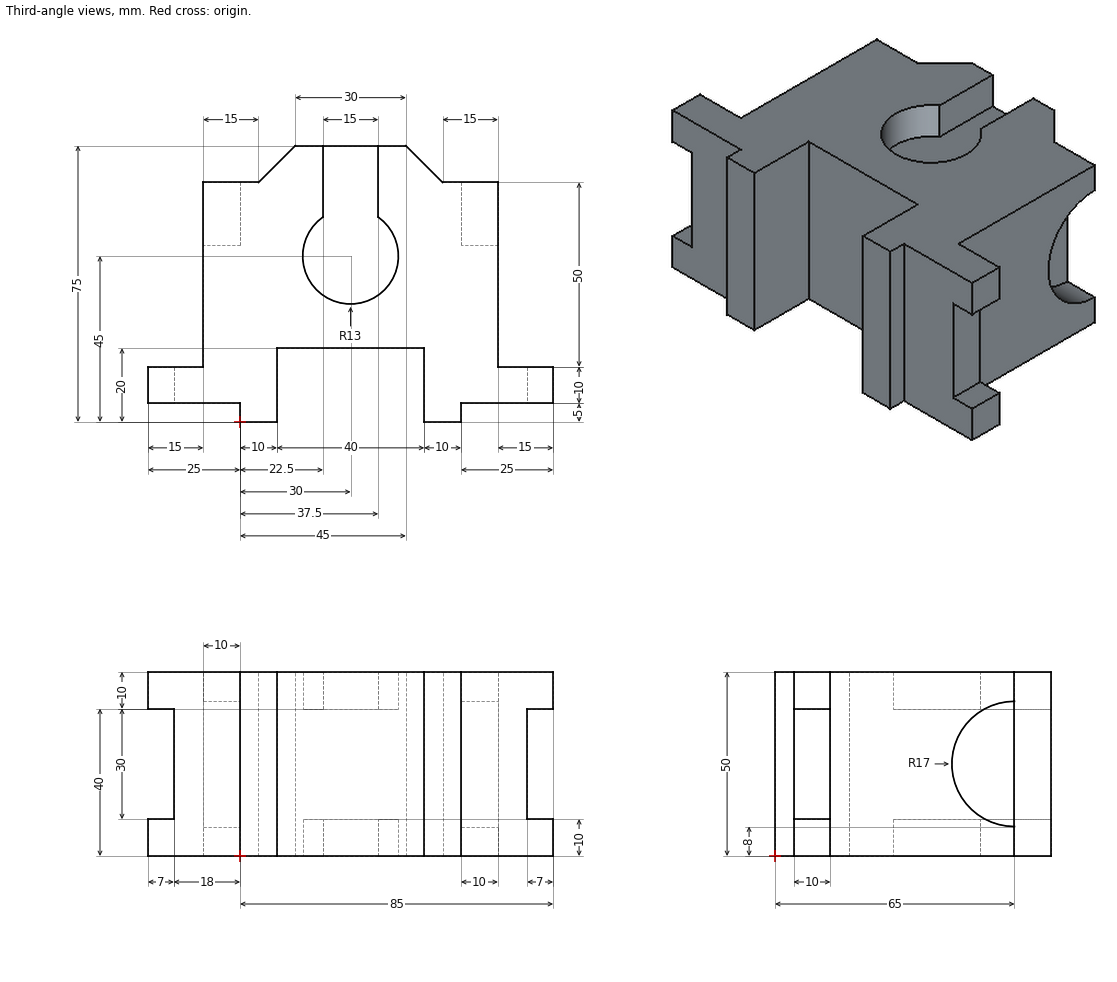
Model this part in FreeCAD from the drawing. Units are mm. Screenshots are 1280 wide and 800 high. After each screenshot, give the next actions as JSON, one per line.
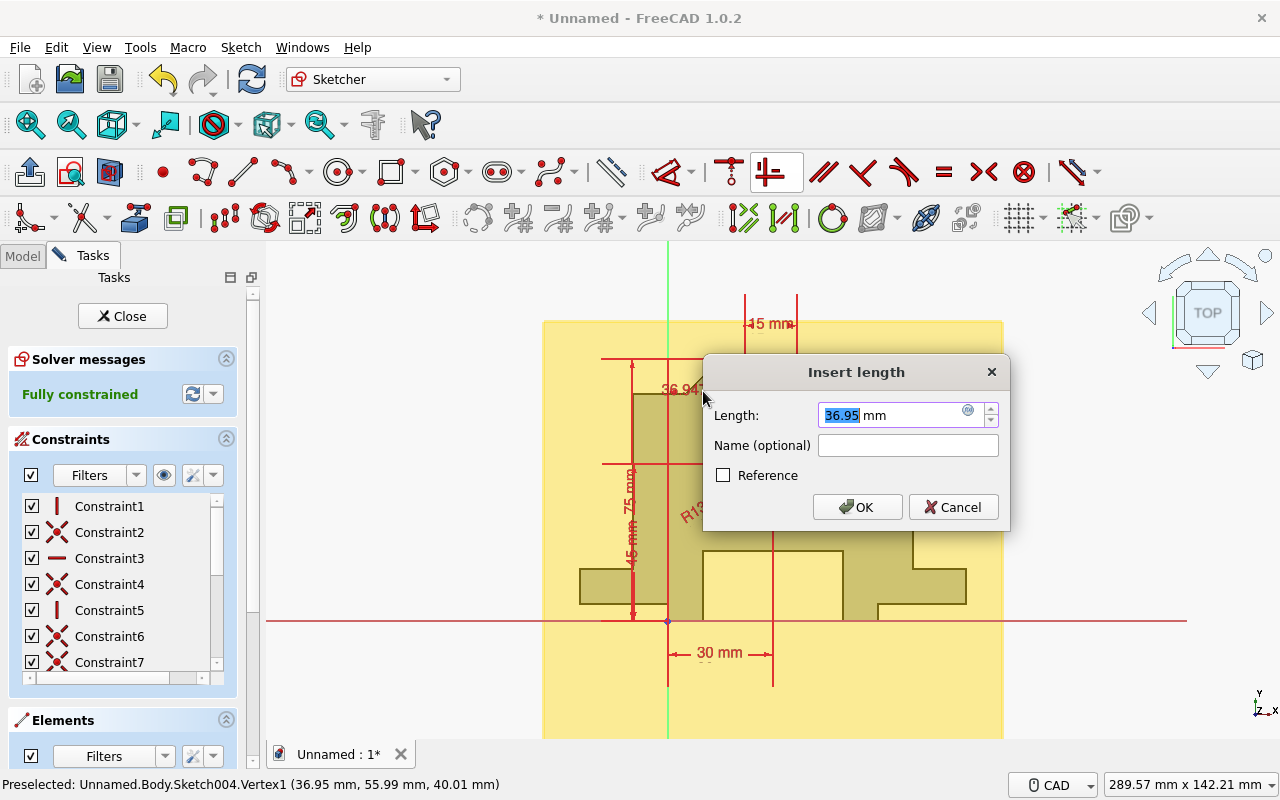
{"action": "type", "text": "37.5"}
{"action": "key", "text": "Return"}
{"action": "key", "text": "Escape"}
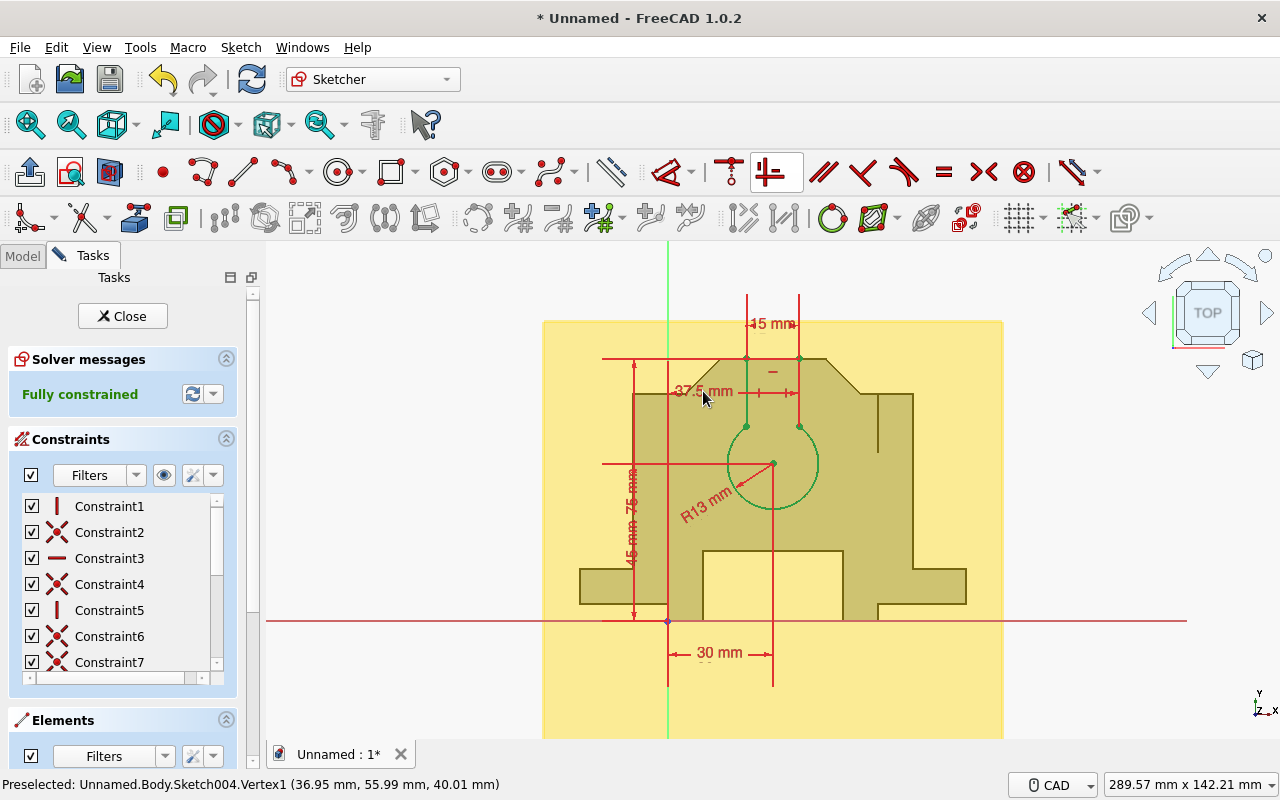
{"action": "left_click", "coordinate": [123, 316]}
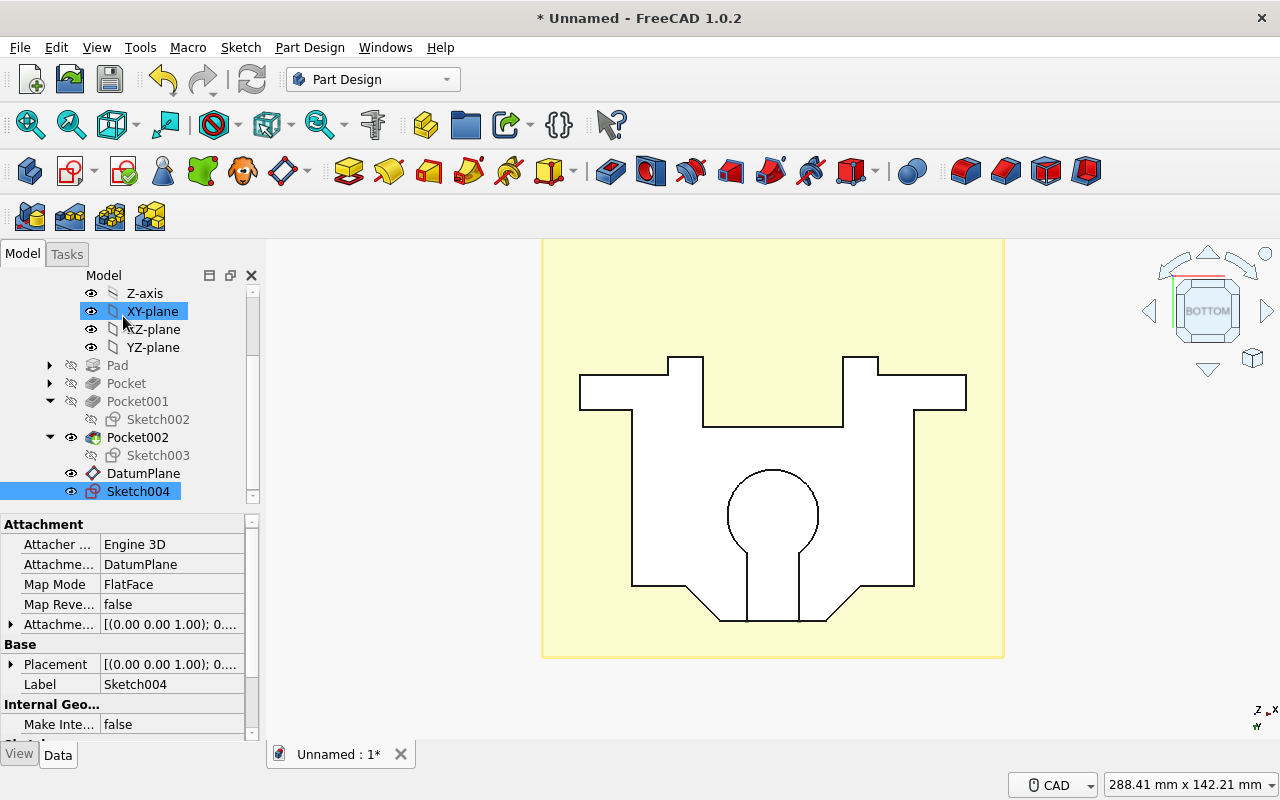
{"action": "left_click", "coordinate": [612, 172]}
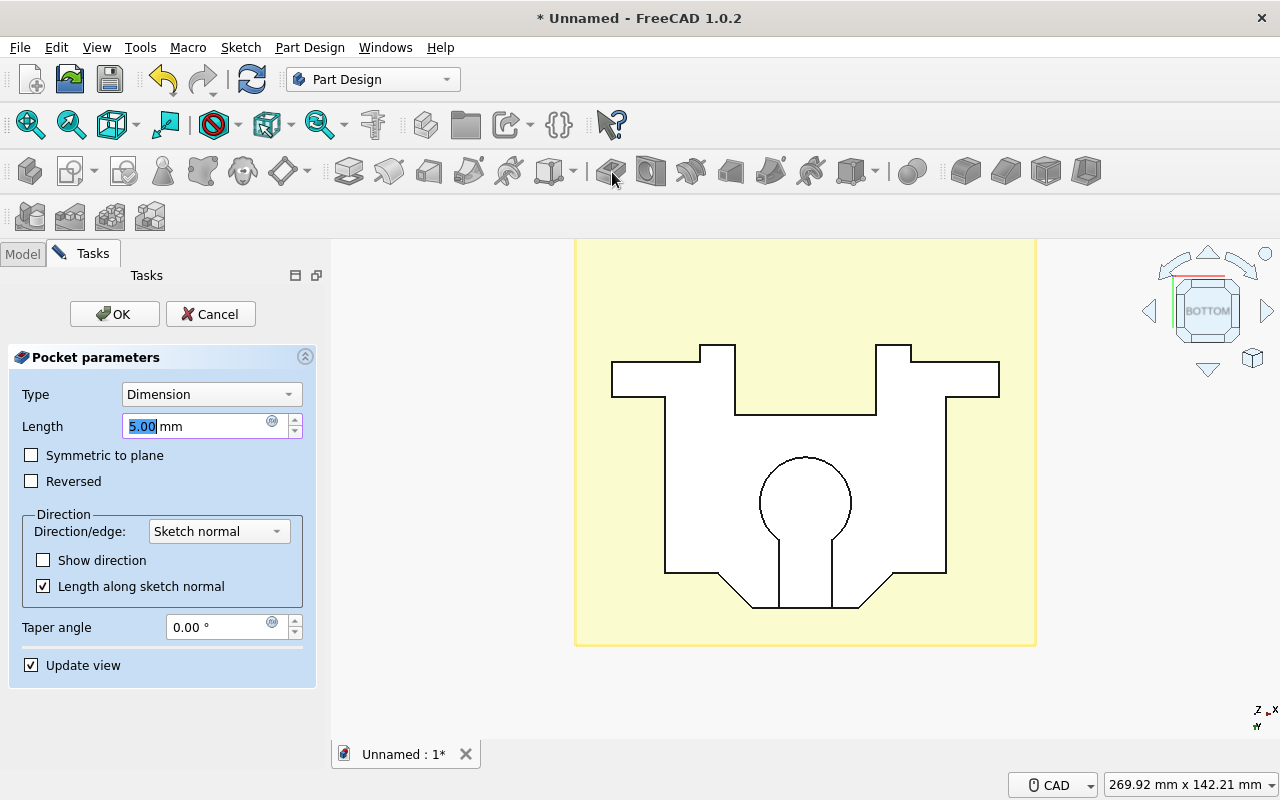
{"action": "type", "text": "10"}
{"action": "key", "text": "Tab"}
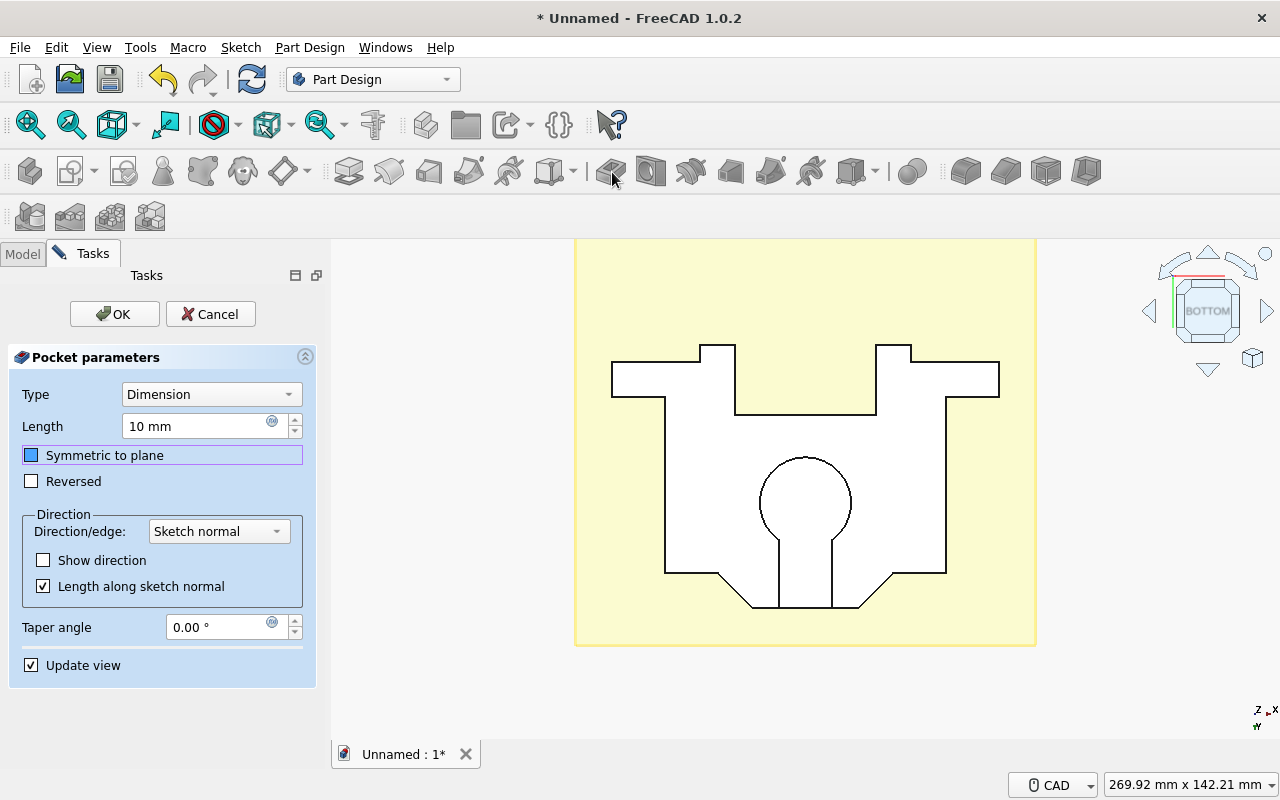
{"action": "left_click", "coordinate": [30, 481]}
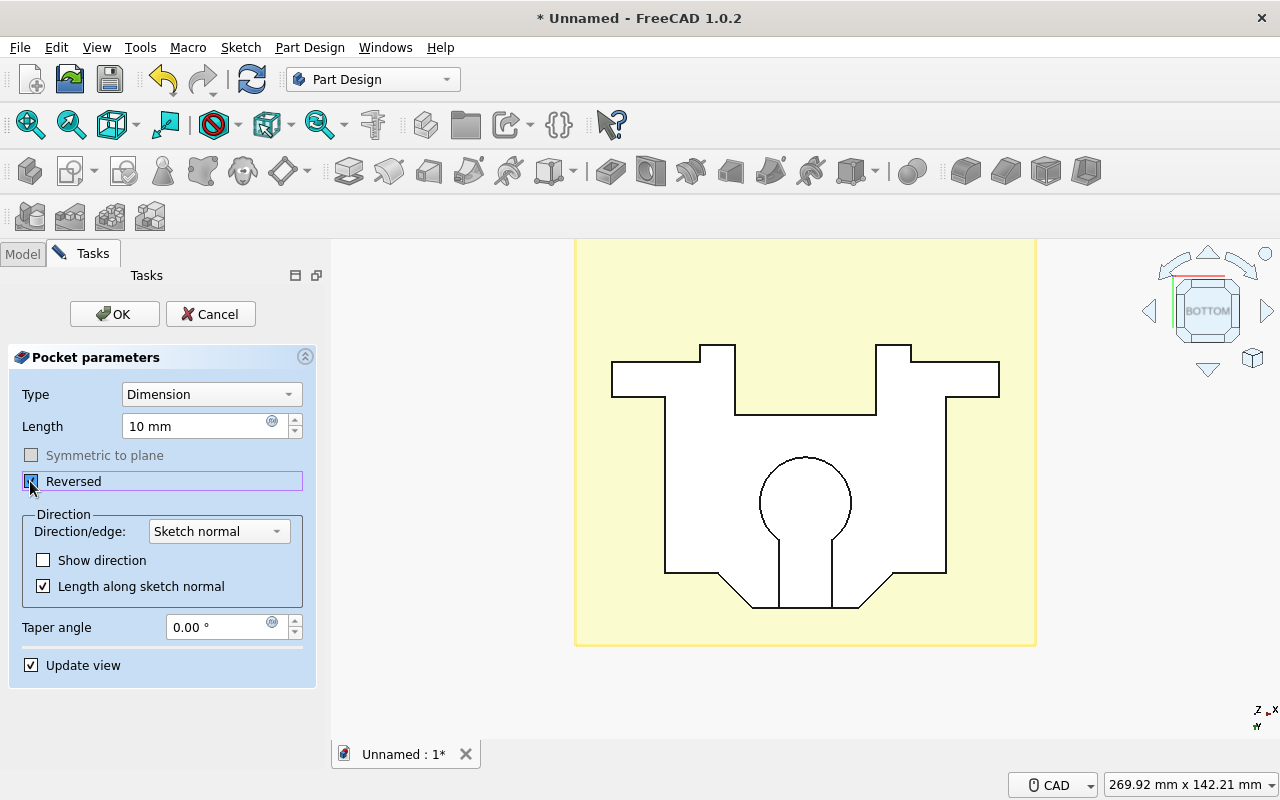
{"action": "left_click", "coordinate": [115, 314]}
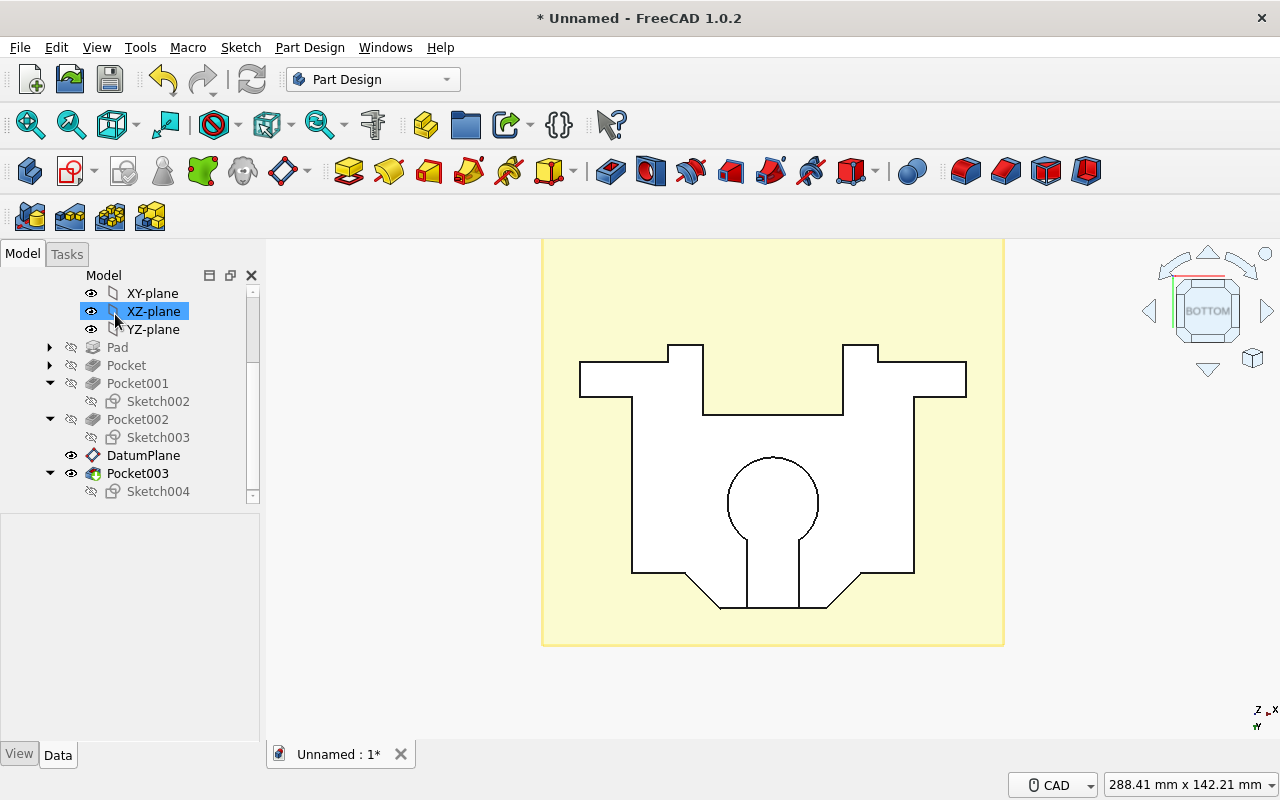
{"action": "left_click", "coordinate": [116, 455]}
{"action": "key", "text": "space"}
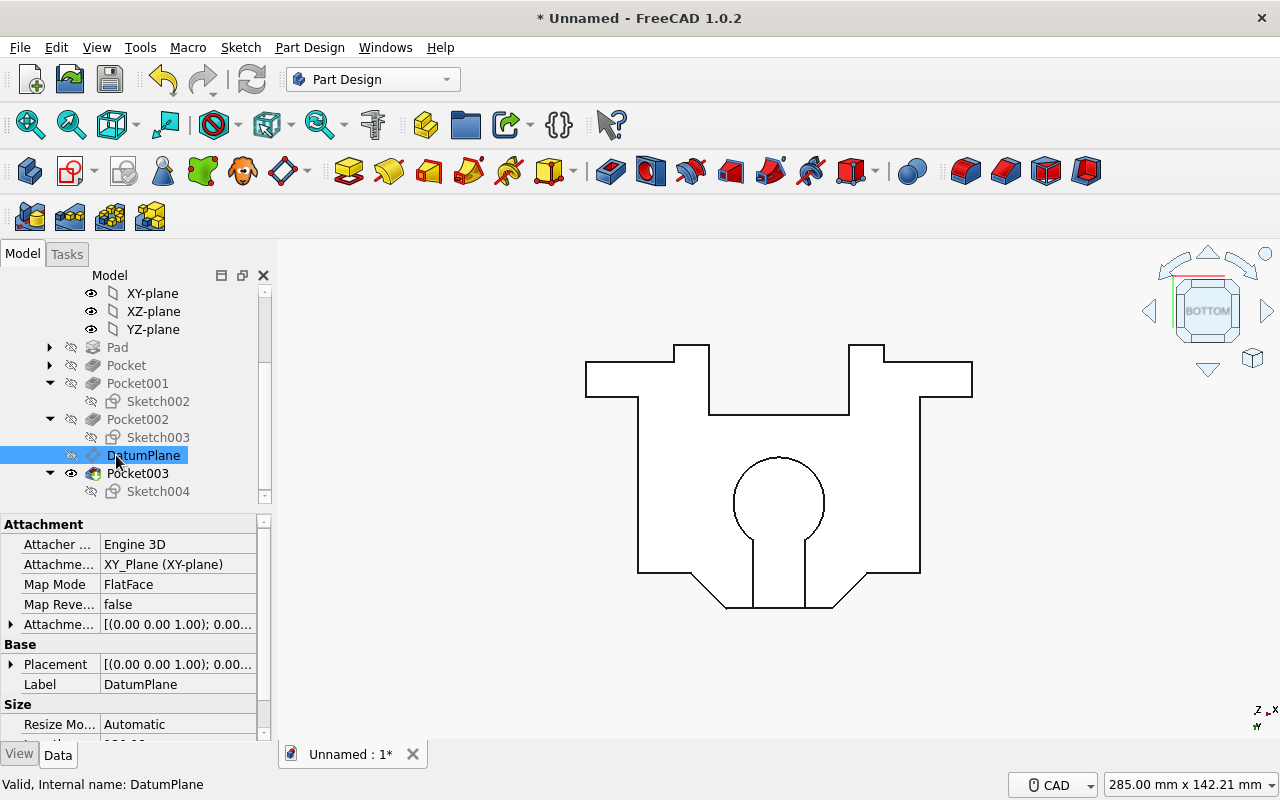
{"action": "key", "text": "4"}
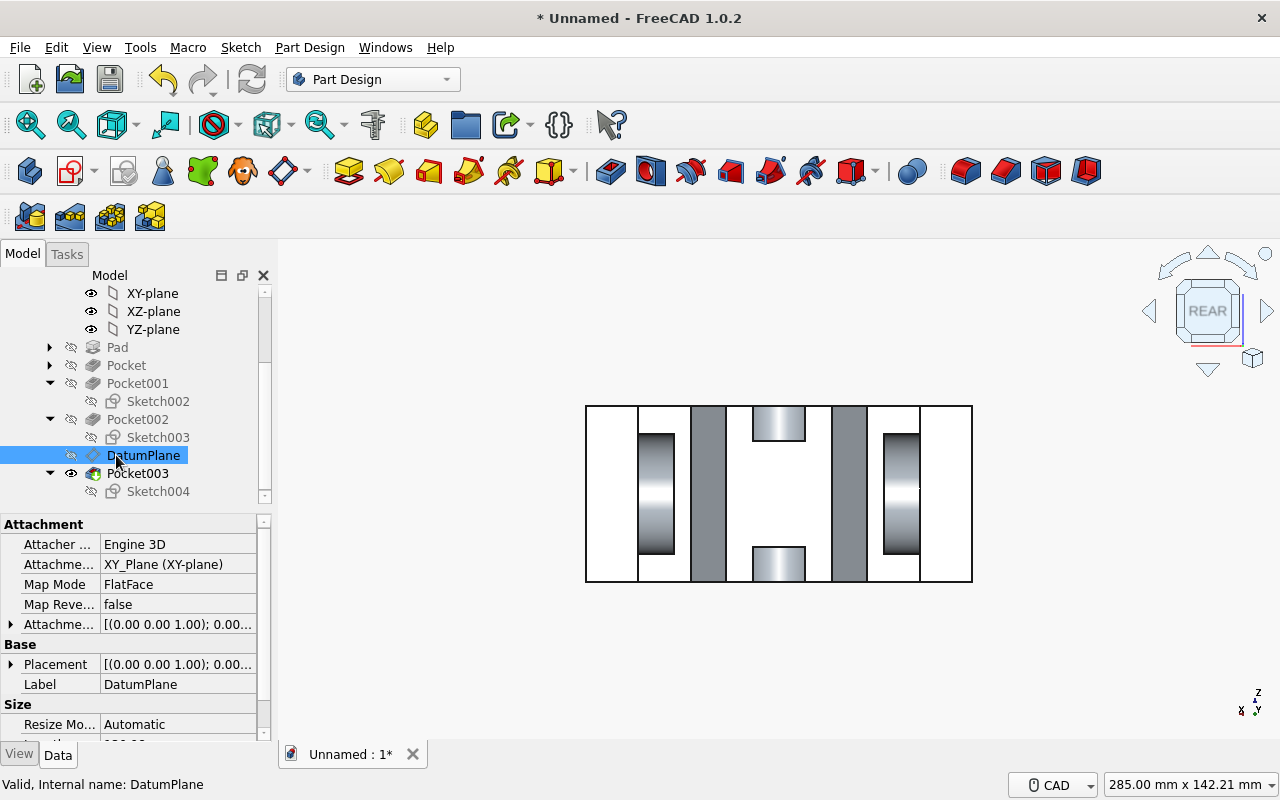
{"action": "left_click", "coordinate": [32, 126]}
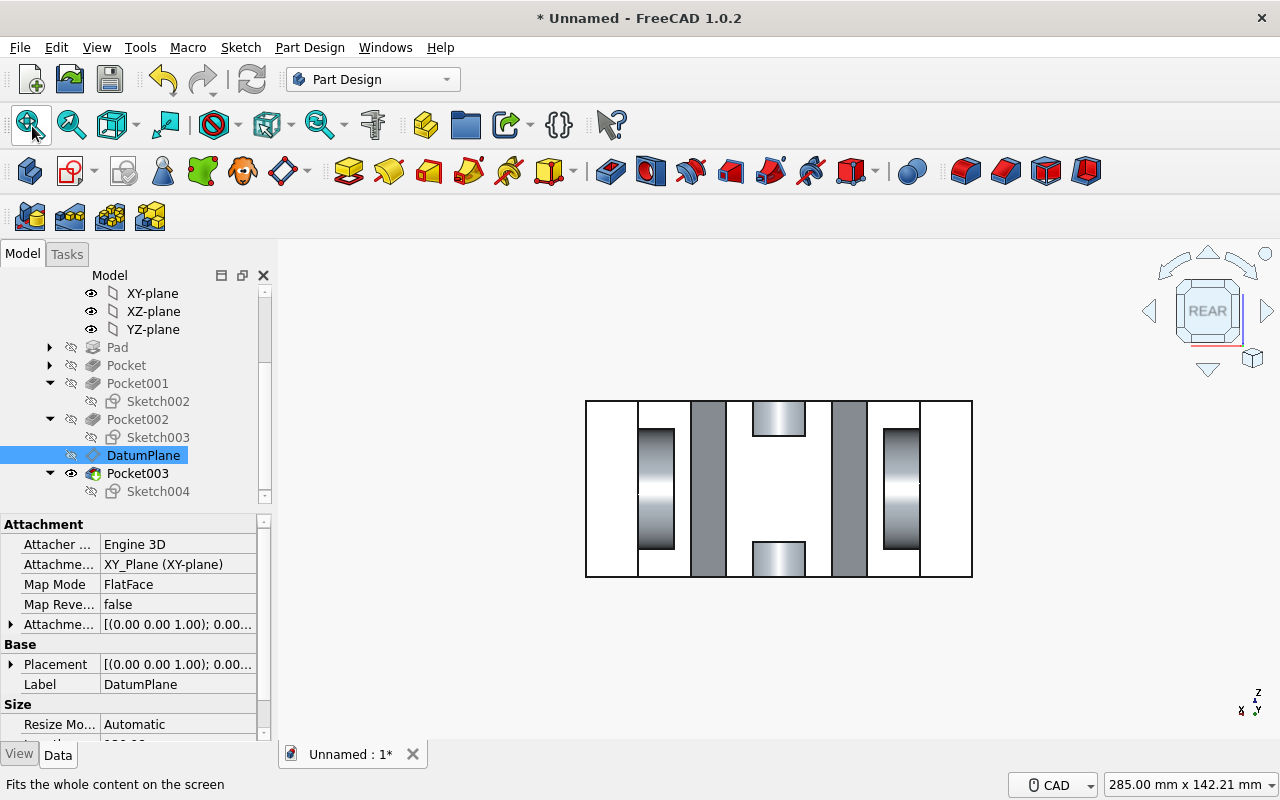
{"action": "left_click", "coordinate": [946, 438]}